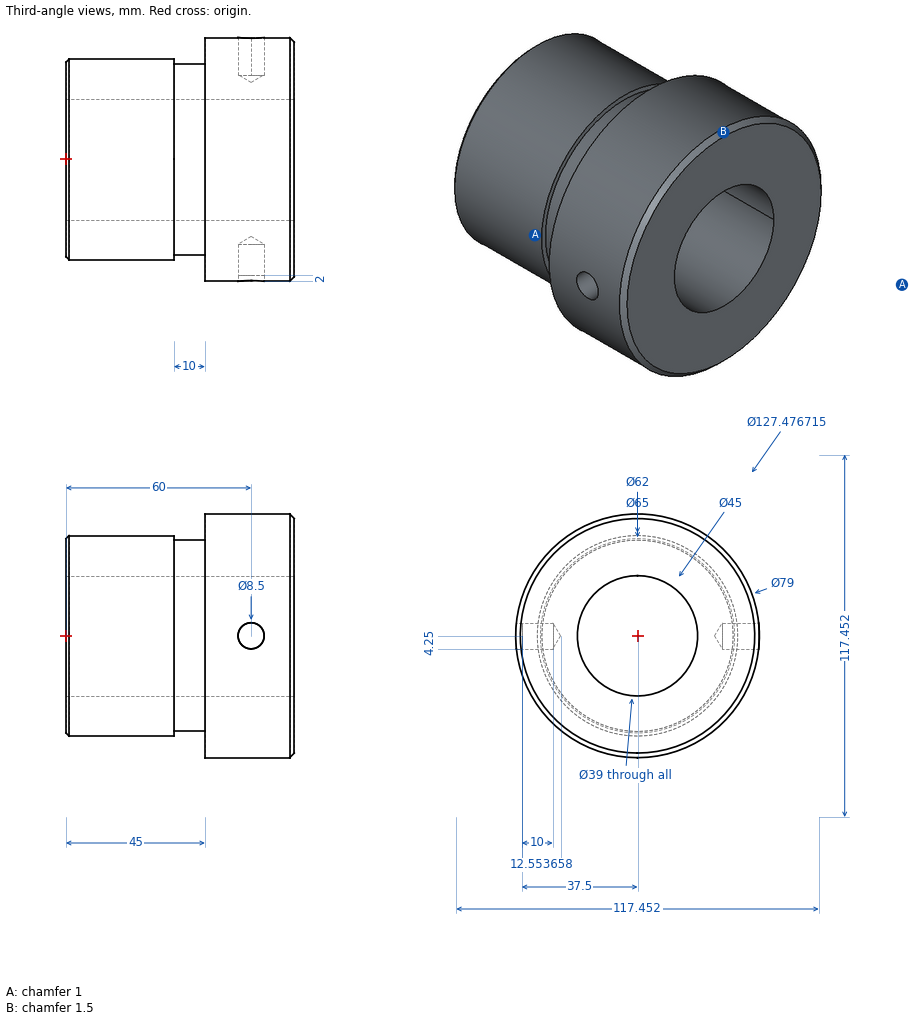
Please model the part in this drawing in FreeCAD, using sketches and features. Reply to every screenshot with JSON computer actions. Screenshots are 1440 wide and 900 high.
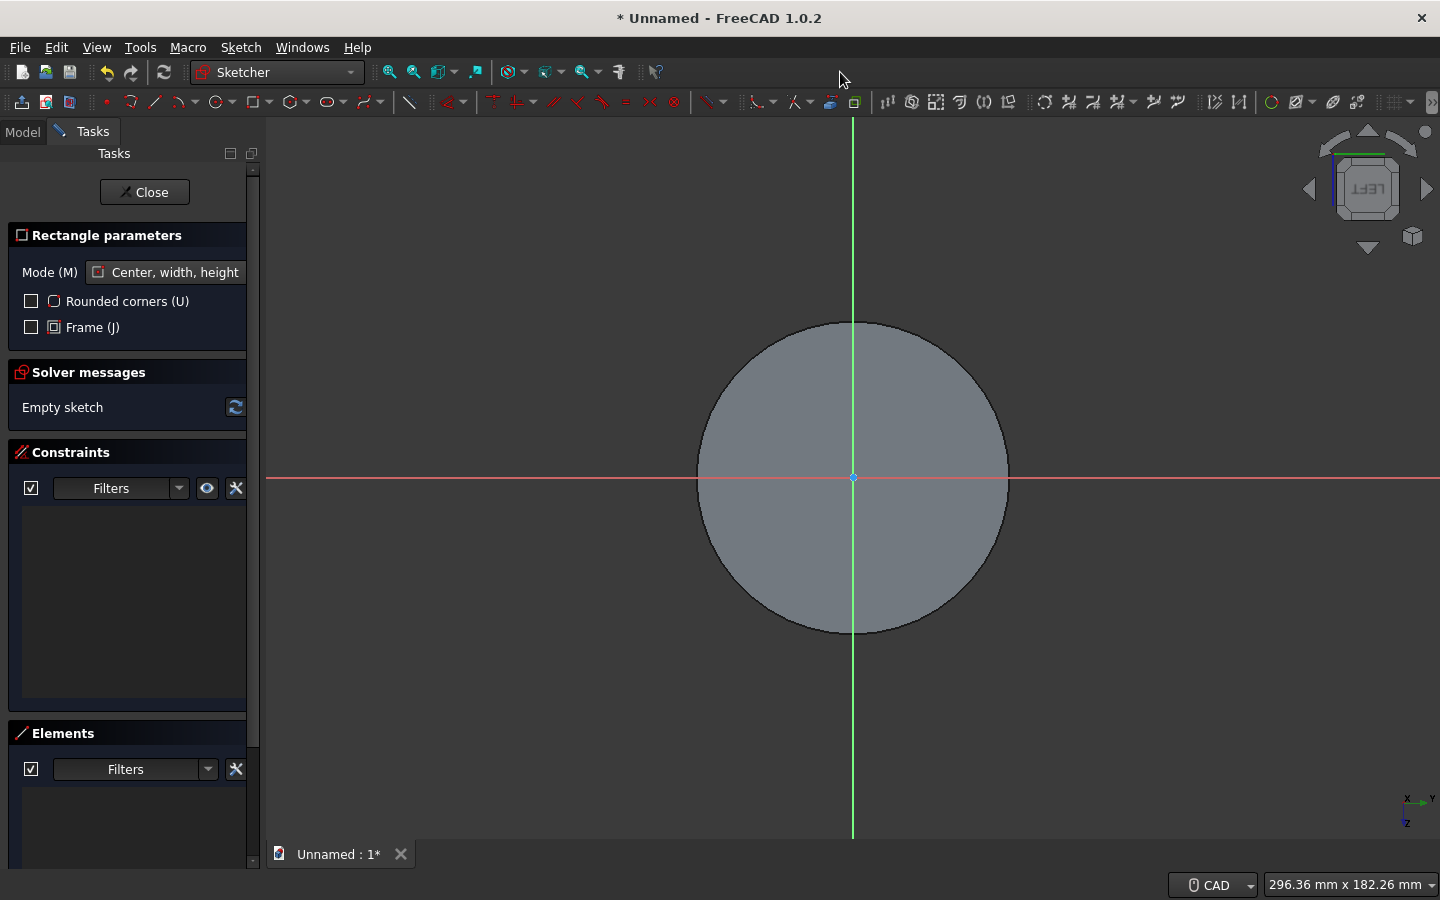
{"action": "left_click", "coordinate": [853, 478]}
{"action": "mouse_move", "coordinate": [1086, 245]}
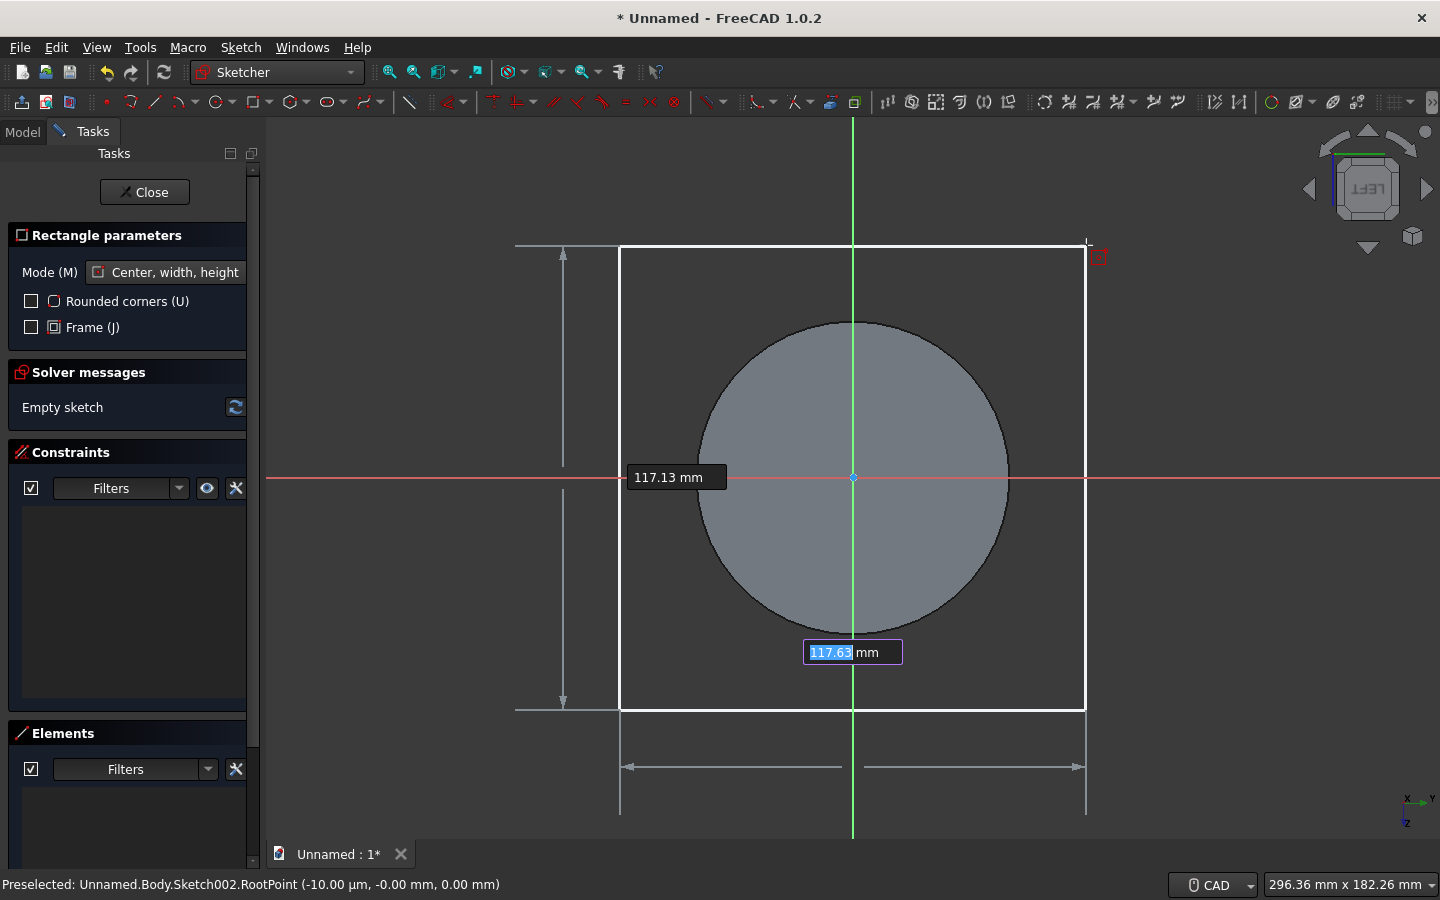
{"action": "type", "text": "117.452"}
{"action": "key", "text": "Tab"}
{"action": "type", "text": "117.452"}
{"action": "key", "text": "Return"}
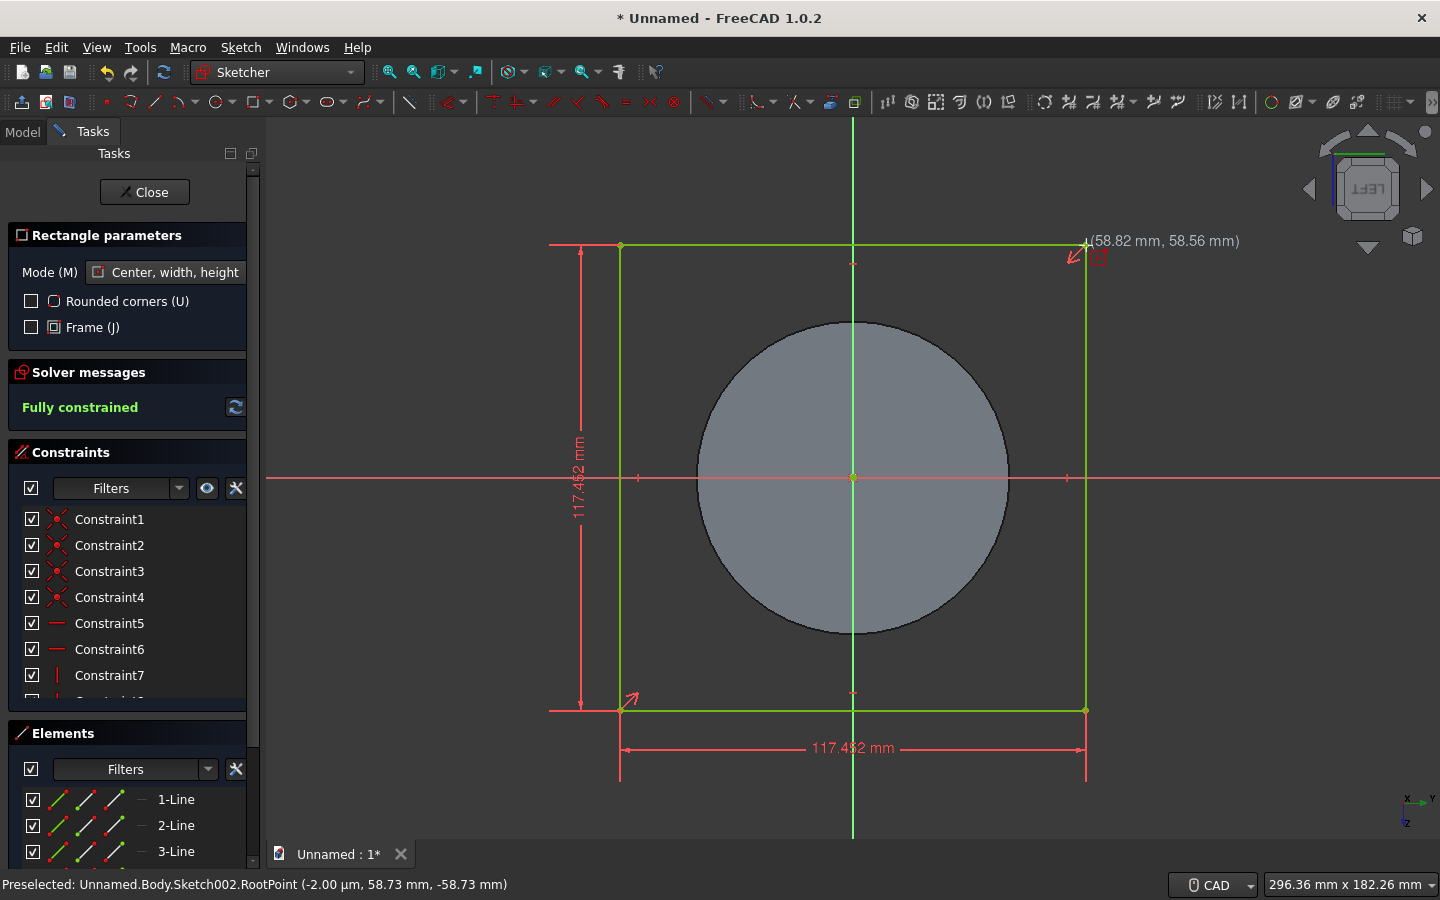
{"action": "key", "text": "g c"}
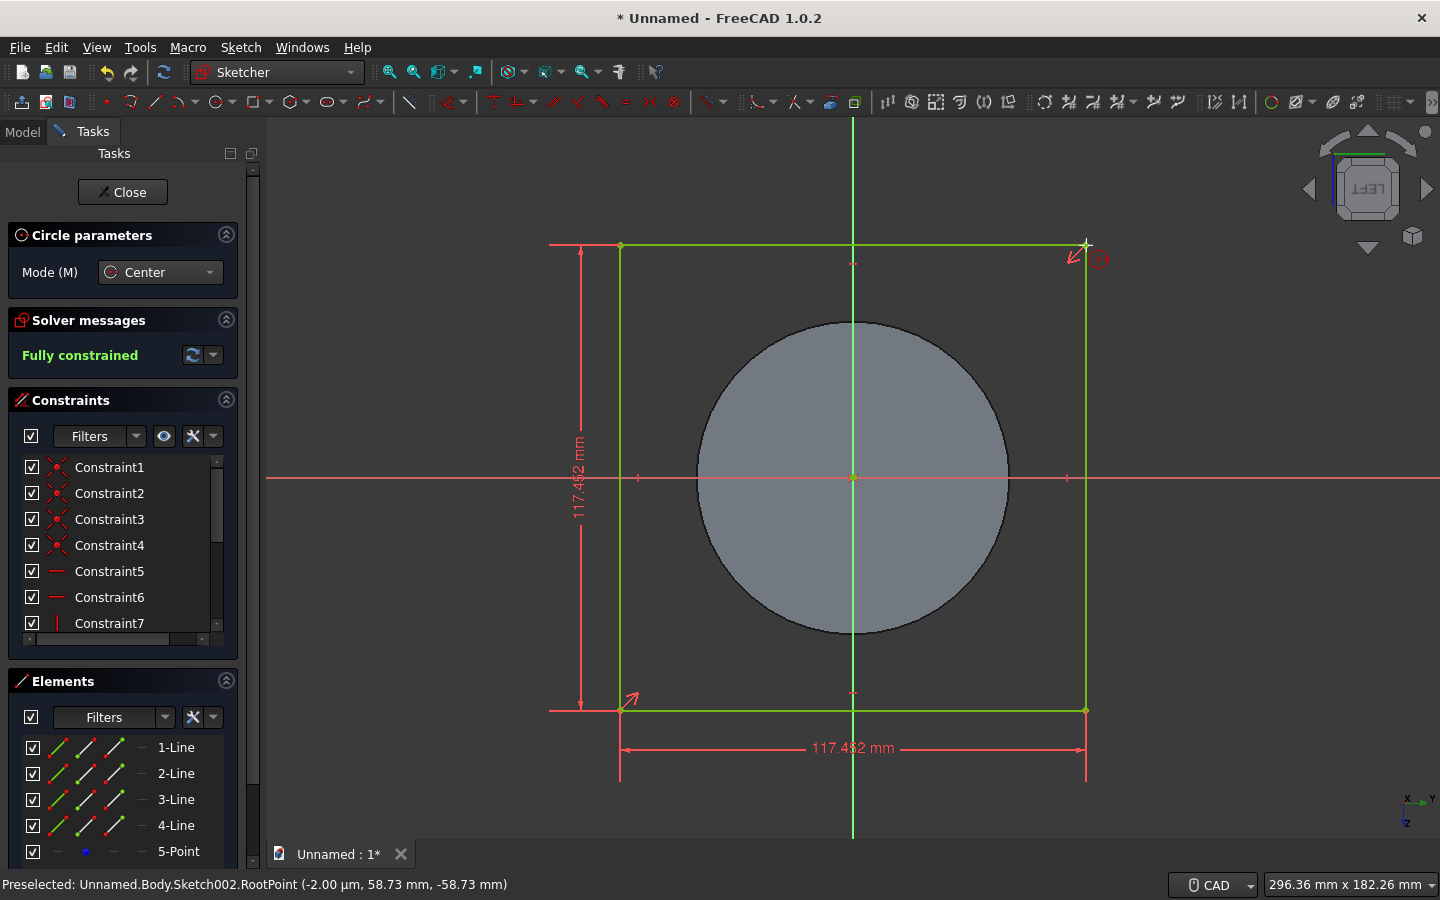
{"action": "left_click", "coordinate": [853, 478]}
{"action": "mouse_move", "coordinate": [944, 387]}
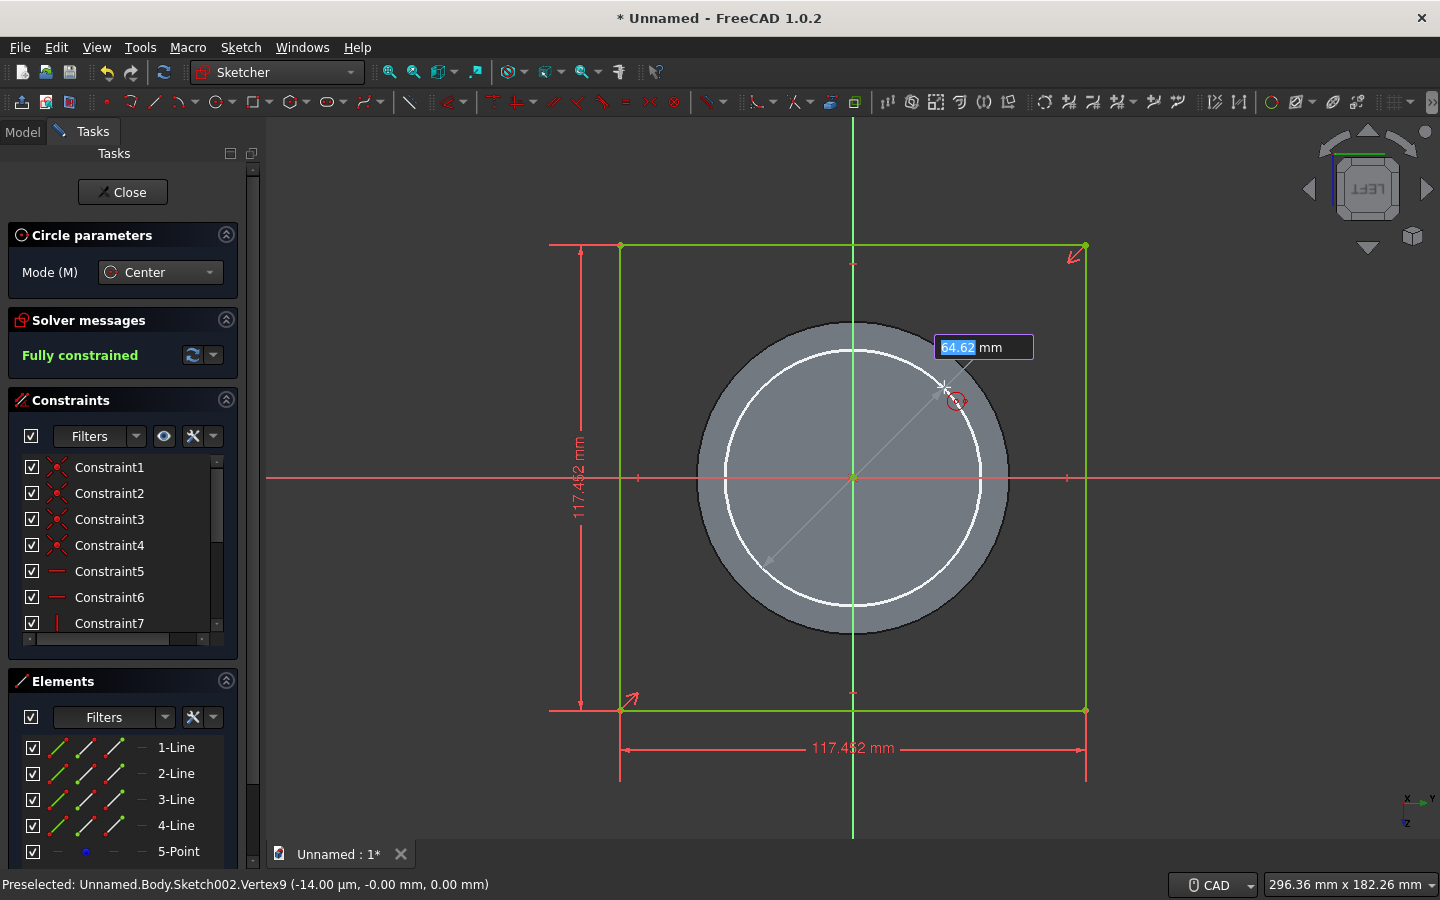
{"action": "type", "text": "65"}
{"action": "key", "text": "Return"}
{"action": "key", "text": "Escape"}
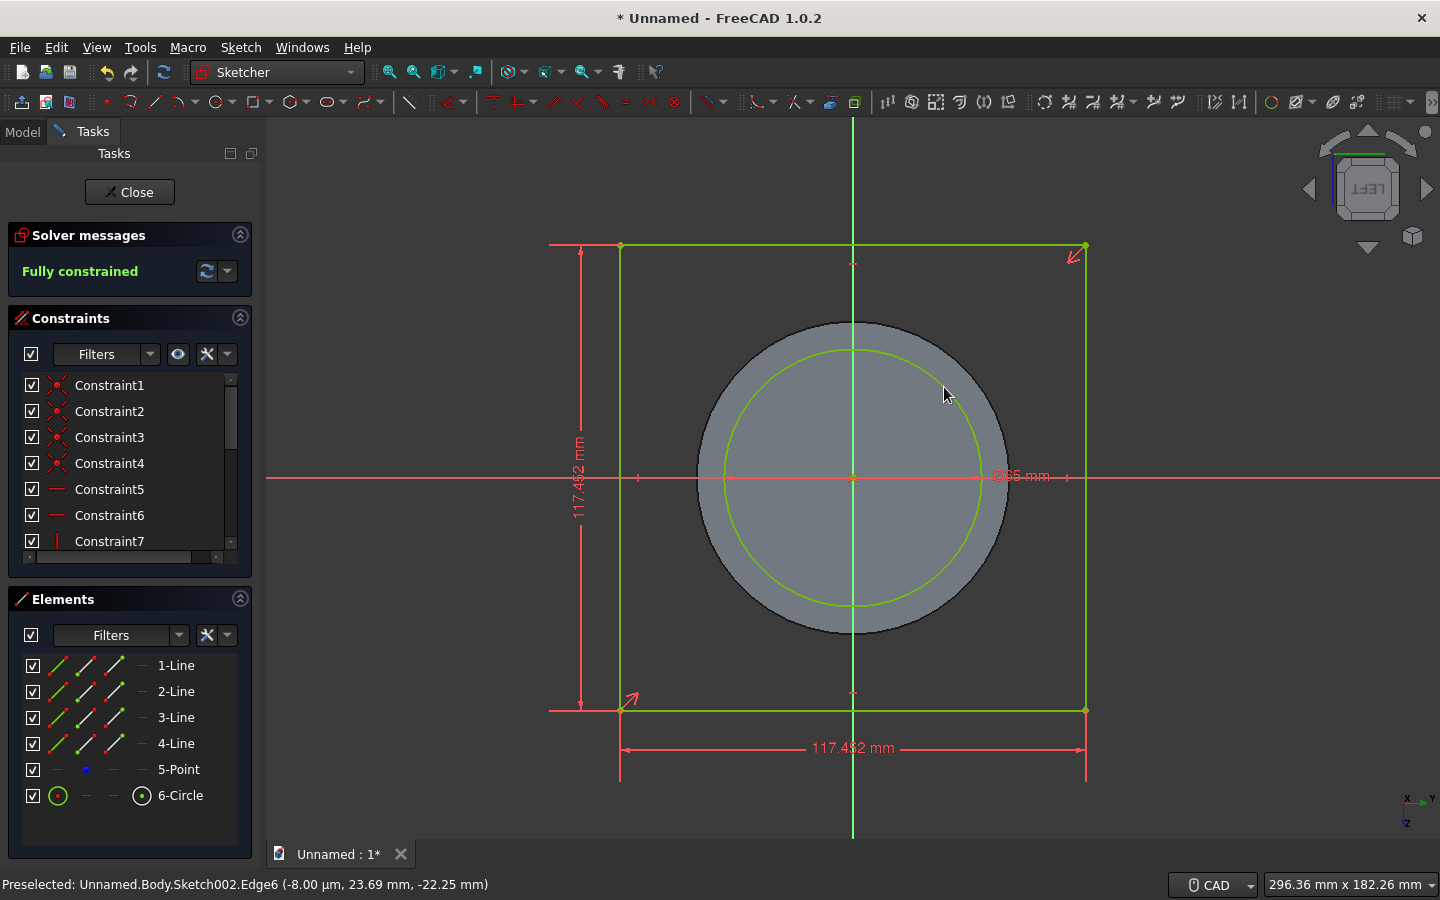
{"action": "left_click", "coordinate": [130, 192]}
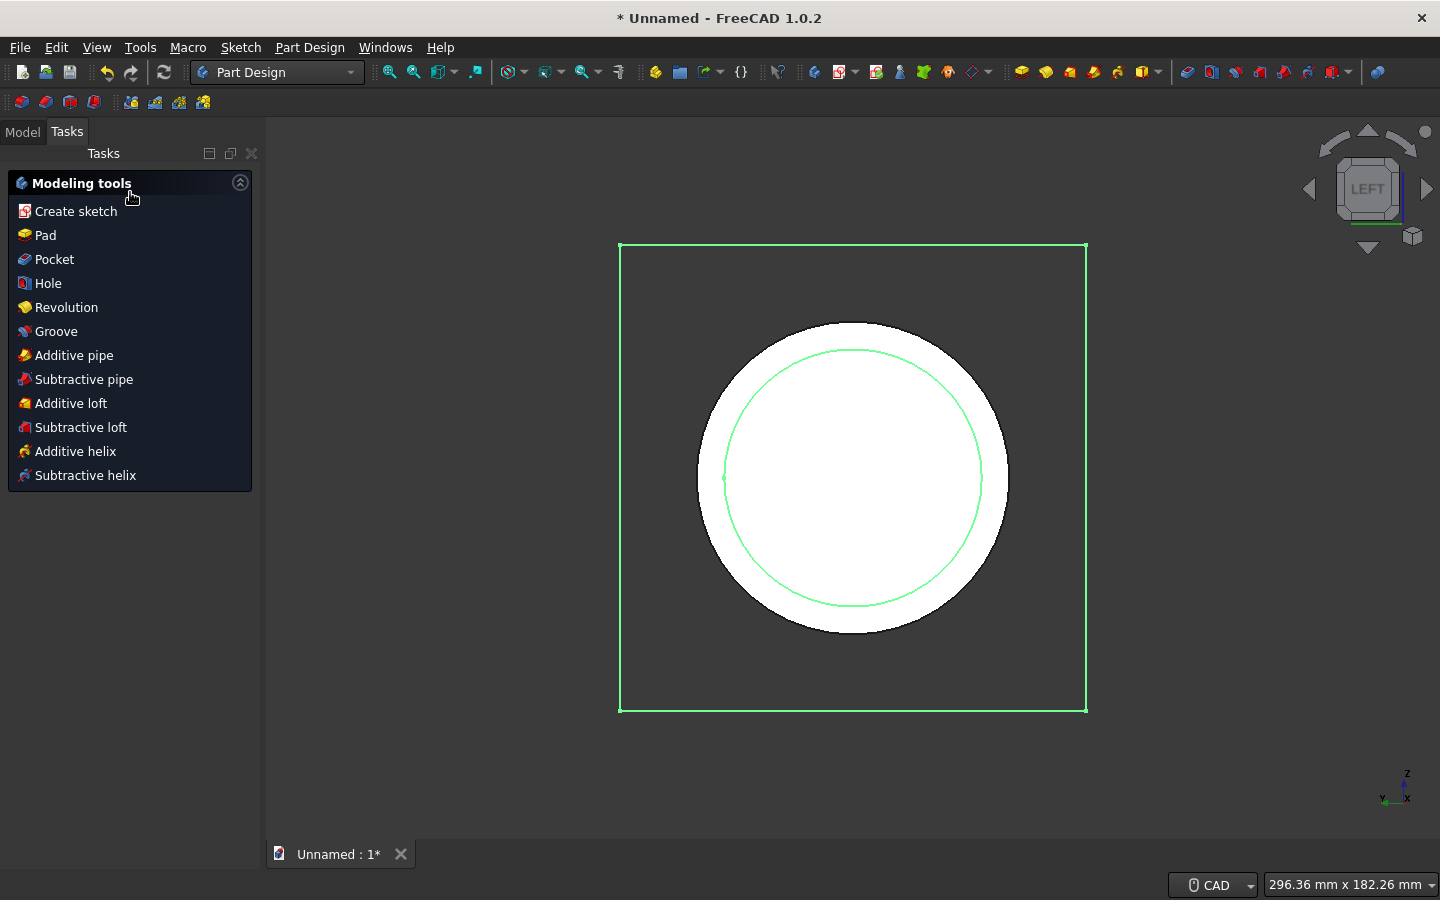
{"action": "left_click", "coordinate": [1188, 72]}